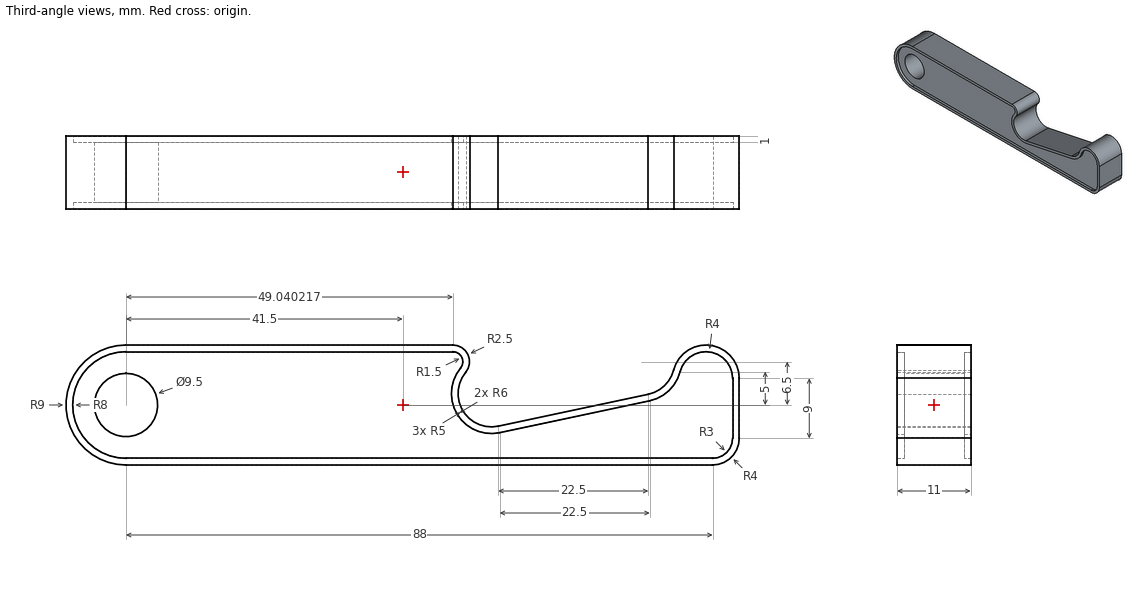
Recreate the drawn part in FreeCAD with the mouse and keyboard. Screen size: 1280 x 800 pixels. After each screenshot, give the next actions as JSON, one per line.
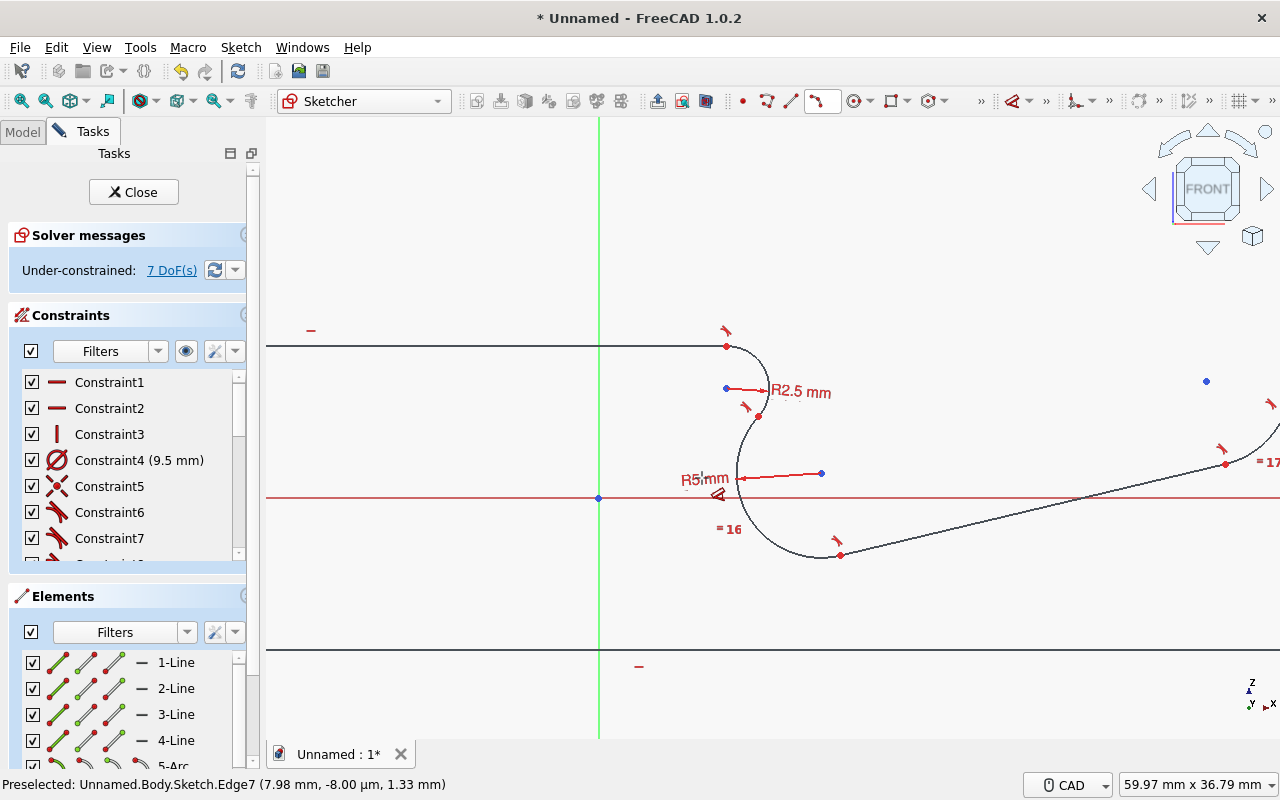
{"action": "scroll", "coordinate": [766, 387], "scroll_direction": "down", "scroll_amount": 5}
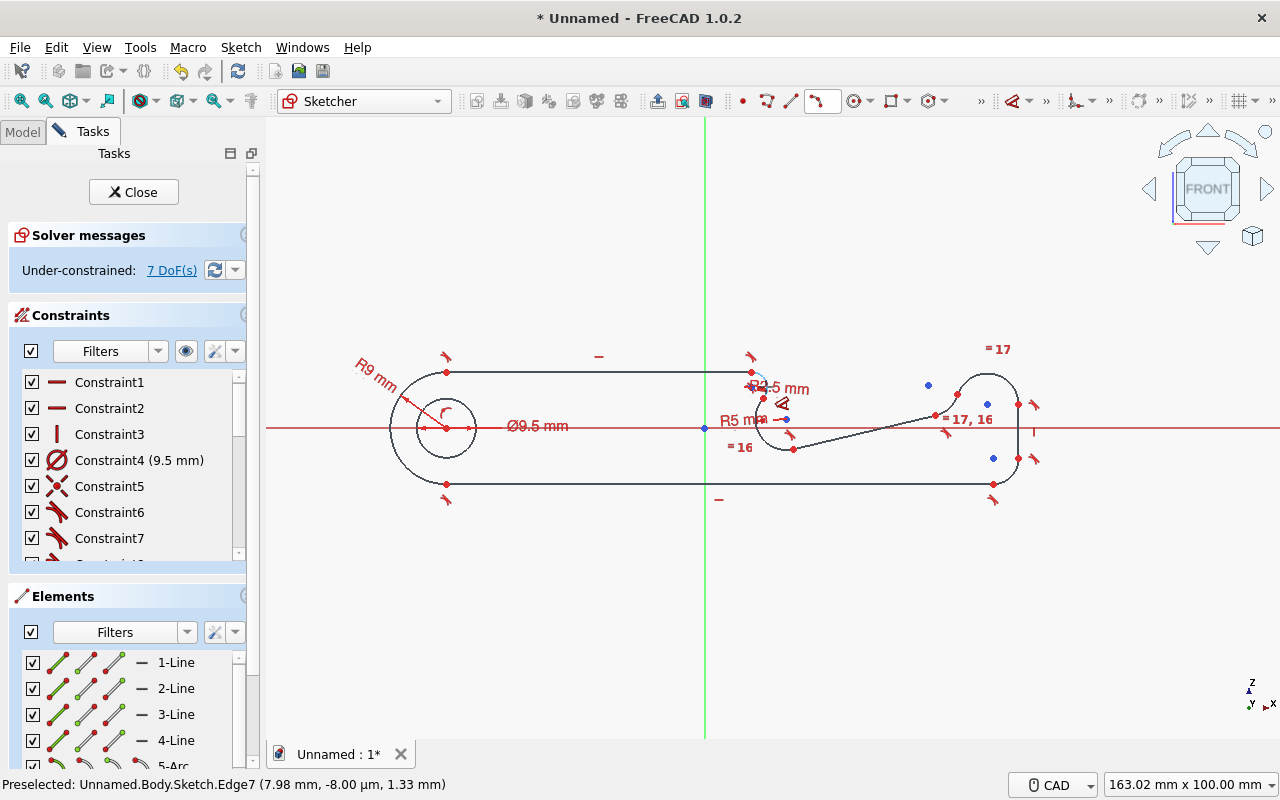
{"action": "scroll", "coordinate": [1005, 481], "scroll_direction": "up", "scroll_amount": 3}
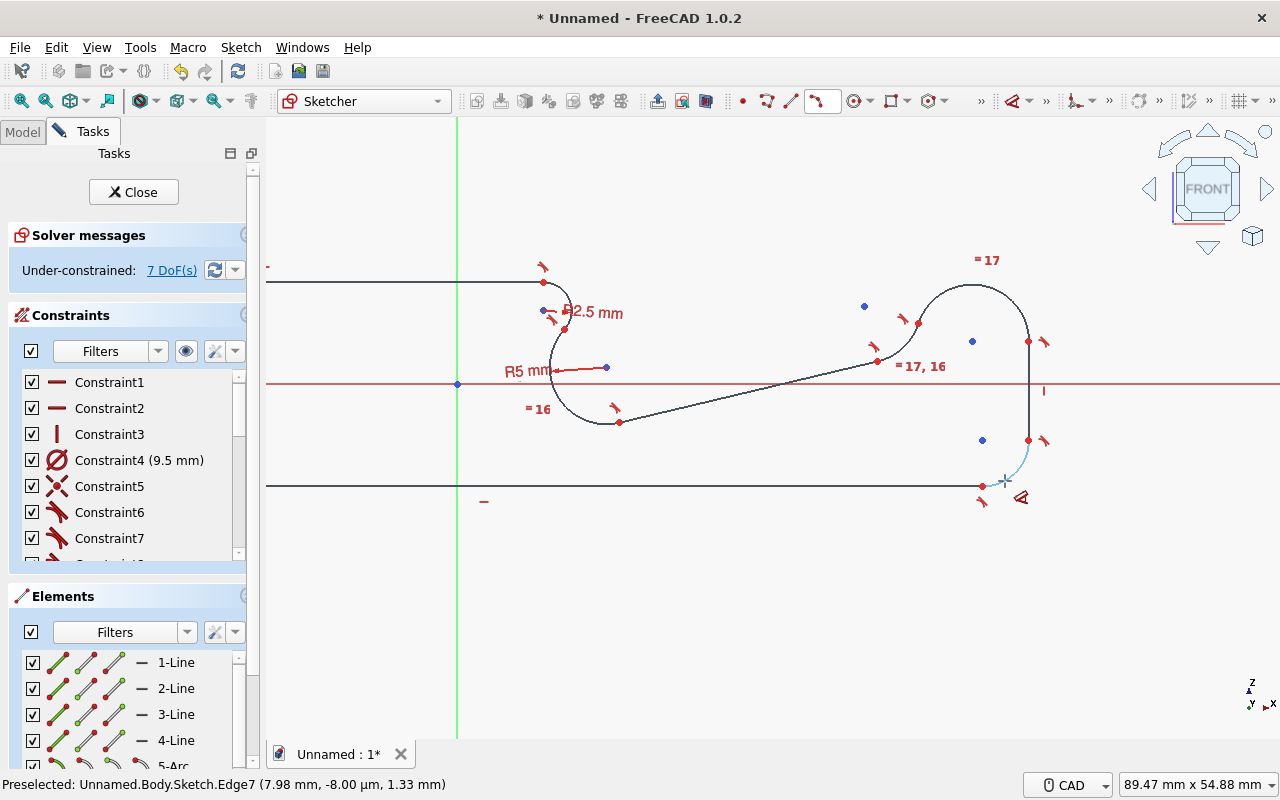
{"action": "left_click", "coordinate": [1004, 481]}
{"action": "left_click", "coordinate": [1019, 509]}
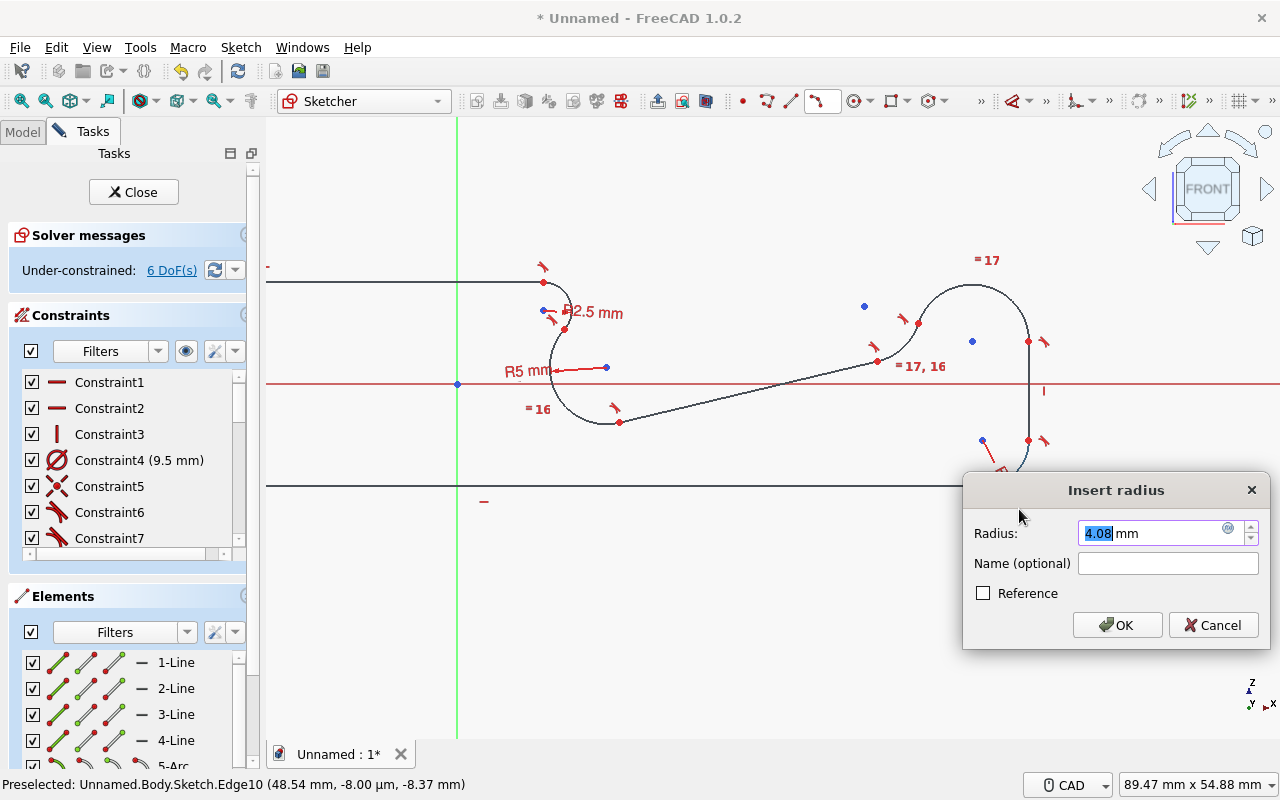
{"action": "type", "text": "4"}
{"action": "key", "text": "Return"}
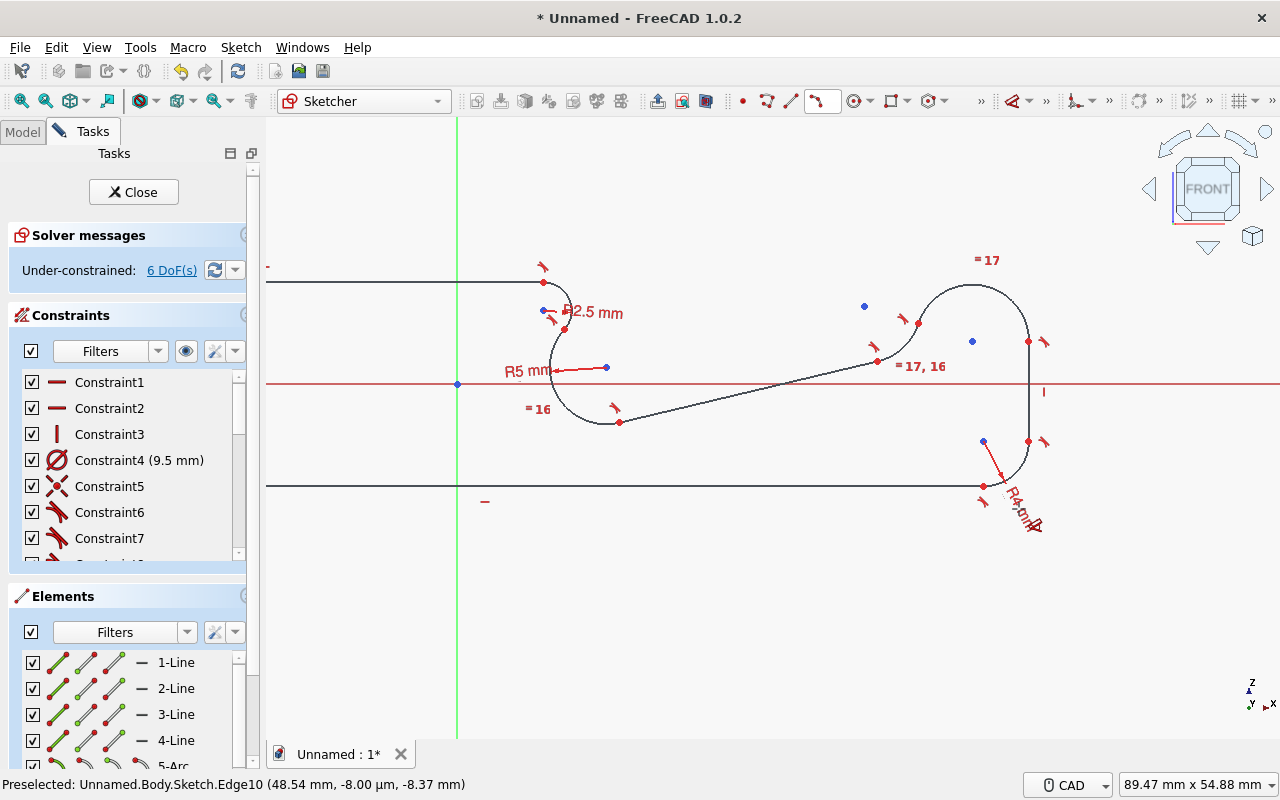
{"action": "left_click", "coordinate": [1029, 371]}
{"action": "left_click", "coordinate": [1063, 368]}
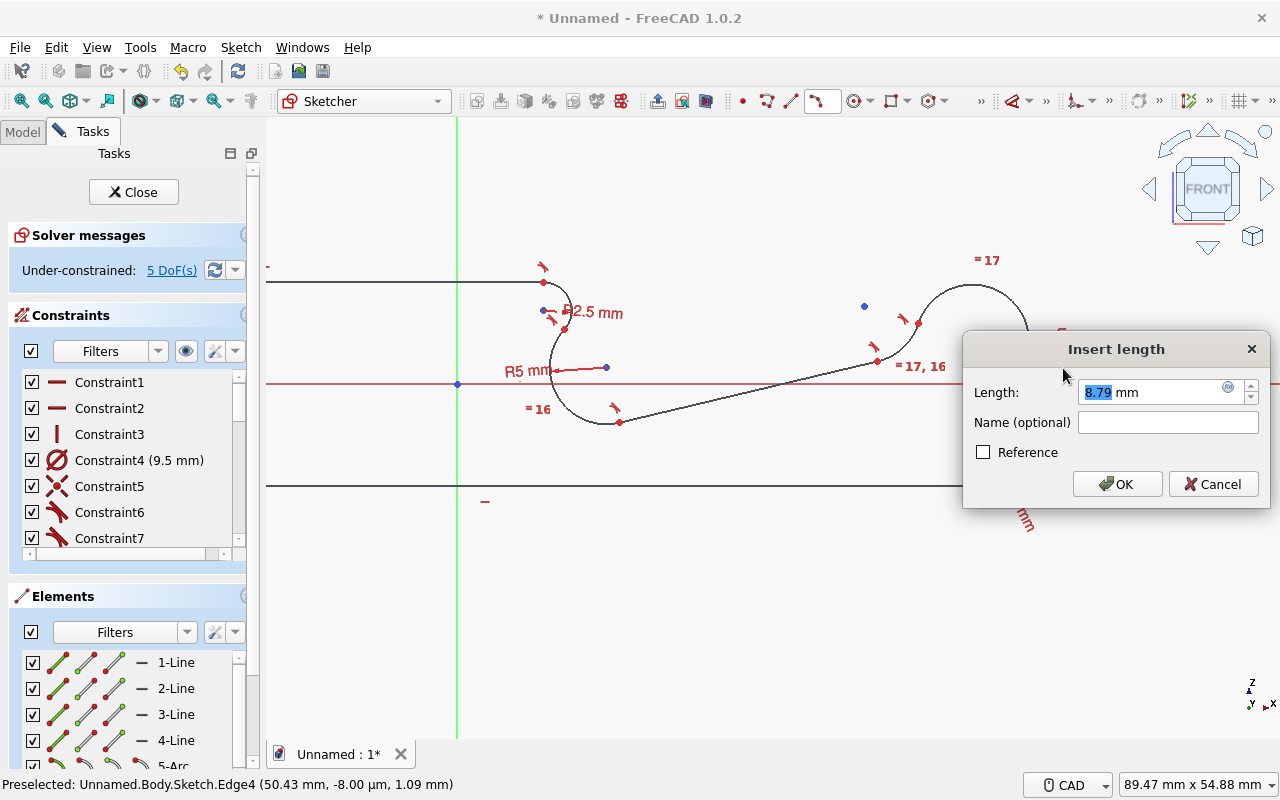
{"action": "type", "text": "9"}
{"action": "key", "text": "Return"}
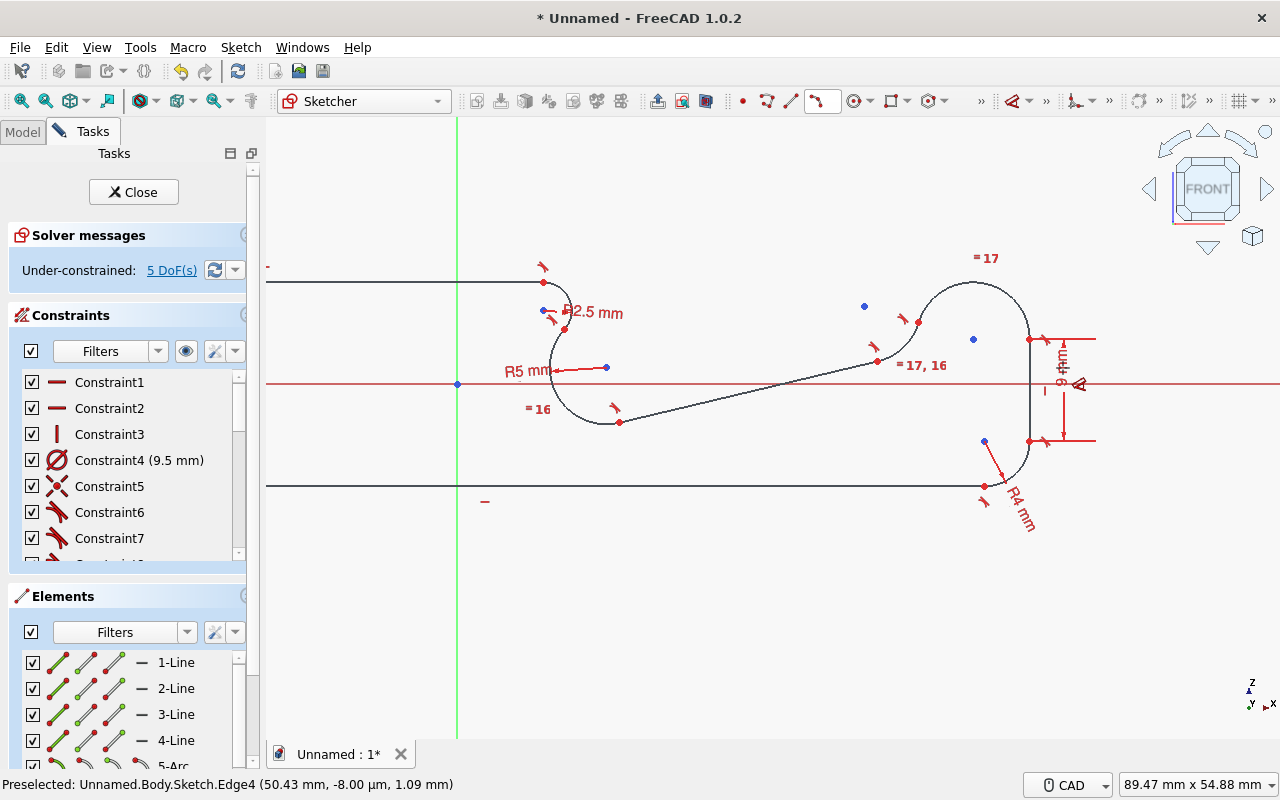
{"action": "left_click", "coordinate": [685, 486]}
{"action": "left_click", "coordinate": [639, 520]}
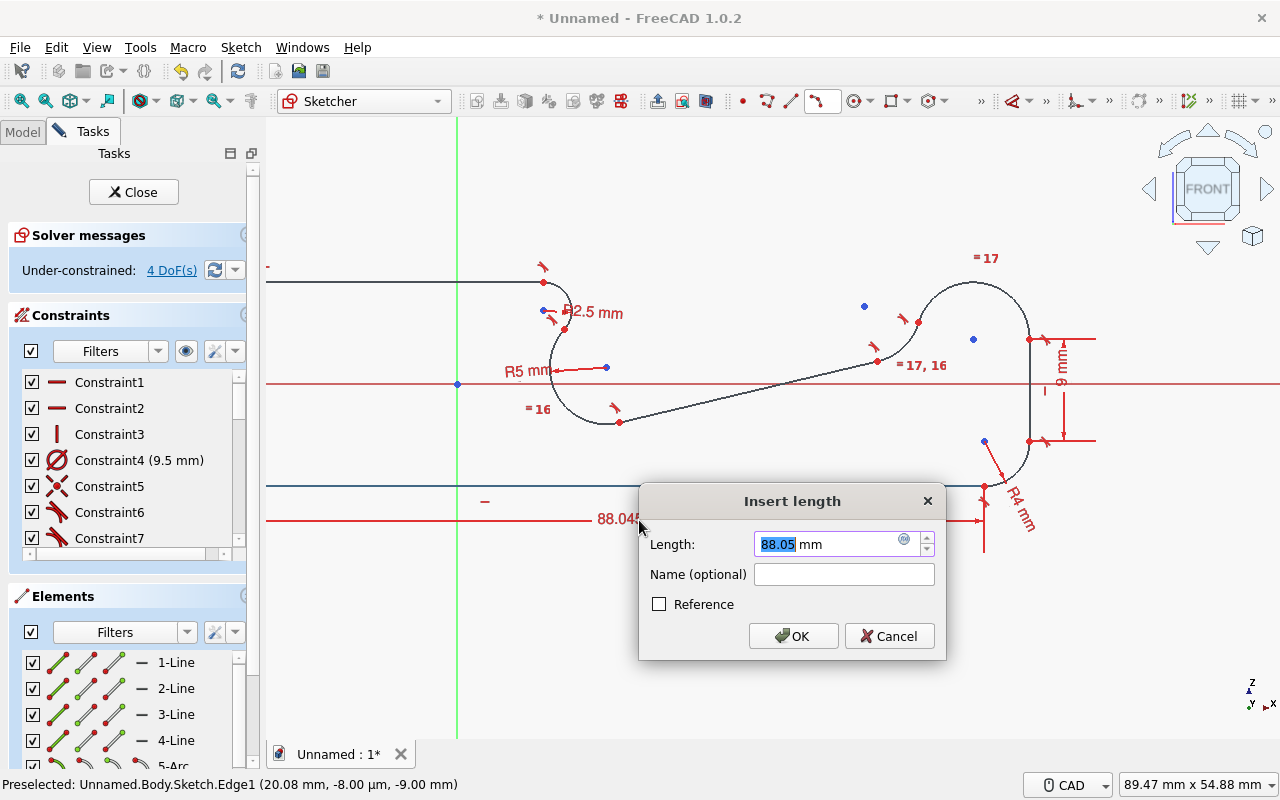
{"action": "type", "text": "88"}
{"action": "key", "text": "Return"}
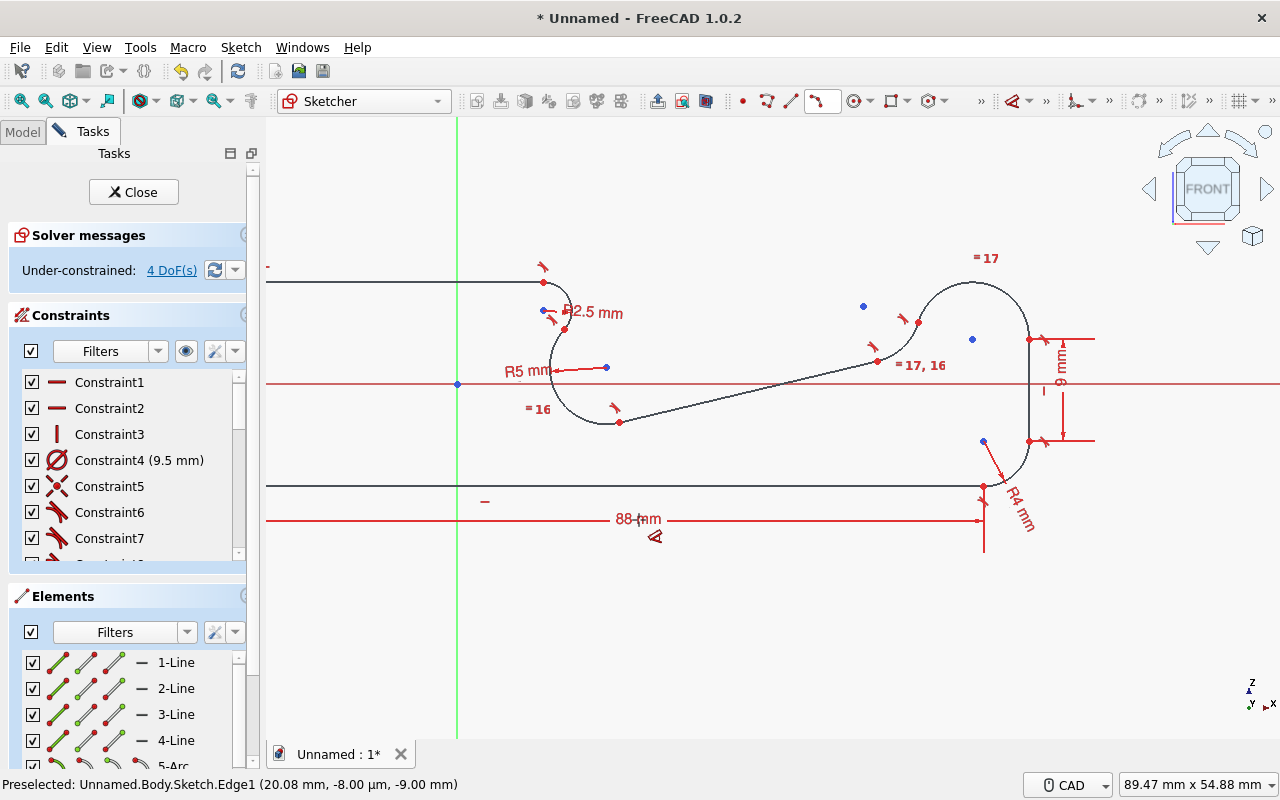
{"action": "left_click", "coordinate": [864, 306]}
{"action": "left_click", "coordinate": [898, 327]}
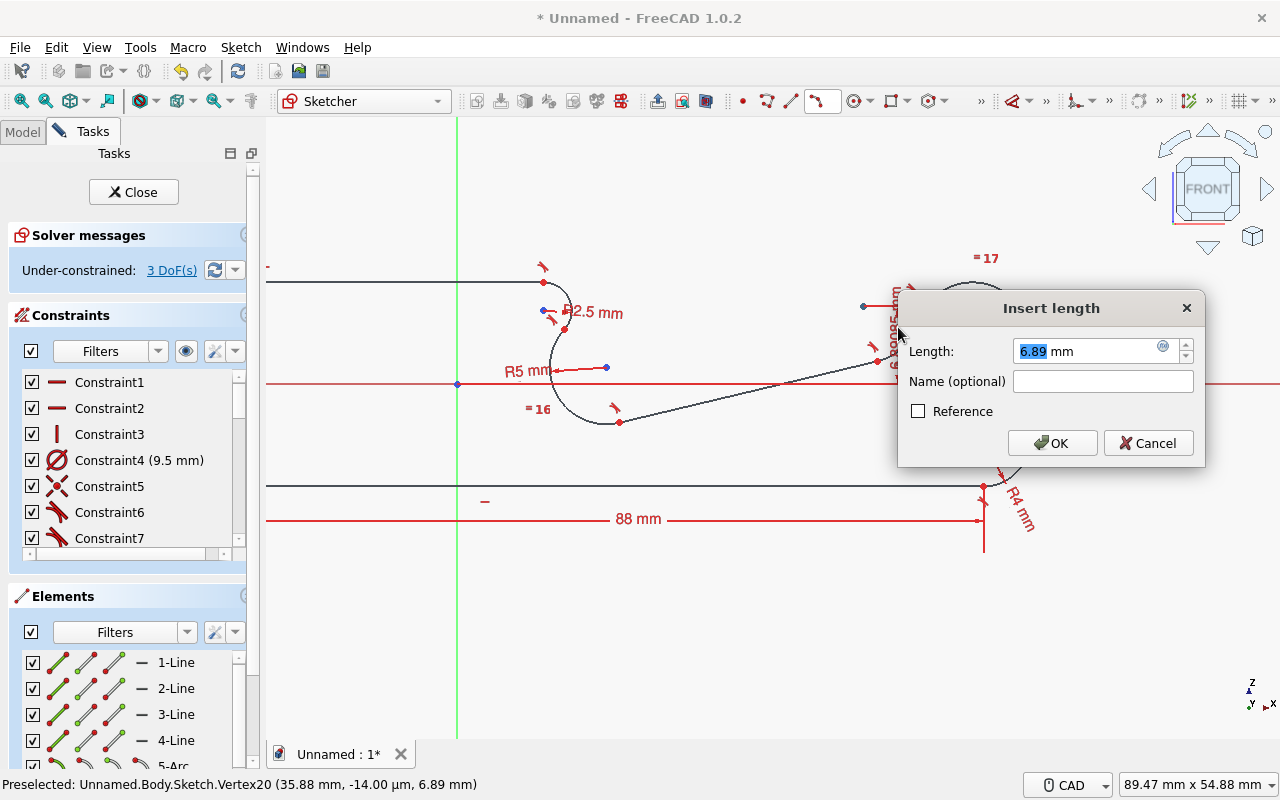
{"action": "type", "text": "6.5"}
{"action": "key", "text": "Return"}